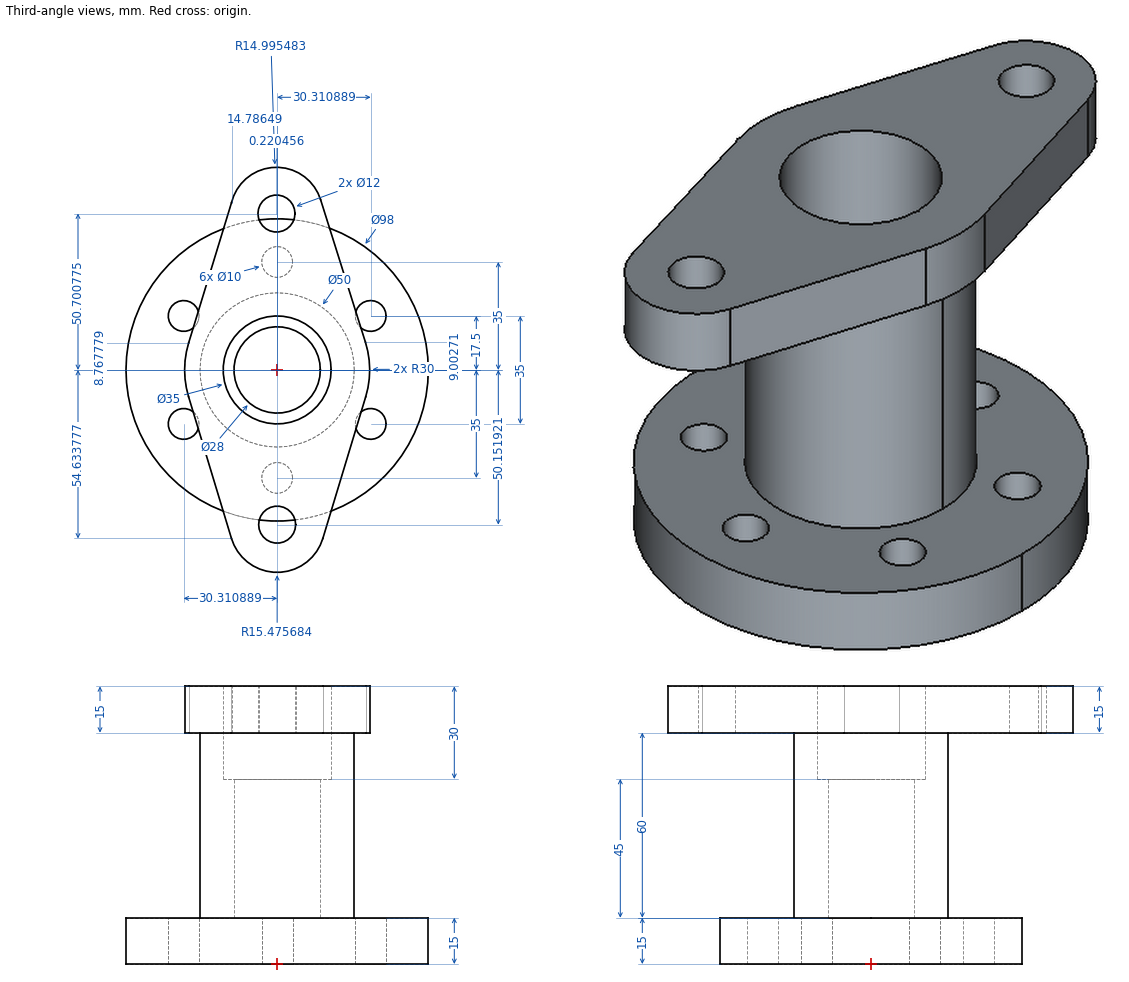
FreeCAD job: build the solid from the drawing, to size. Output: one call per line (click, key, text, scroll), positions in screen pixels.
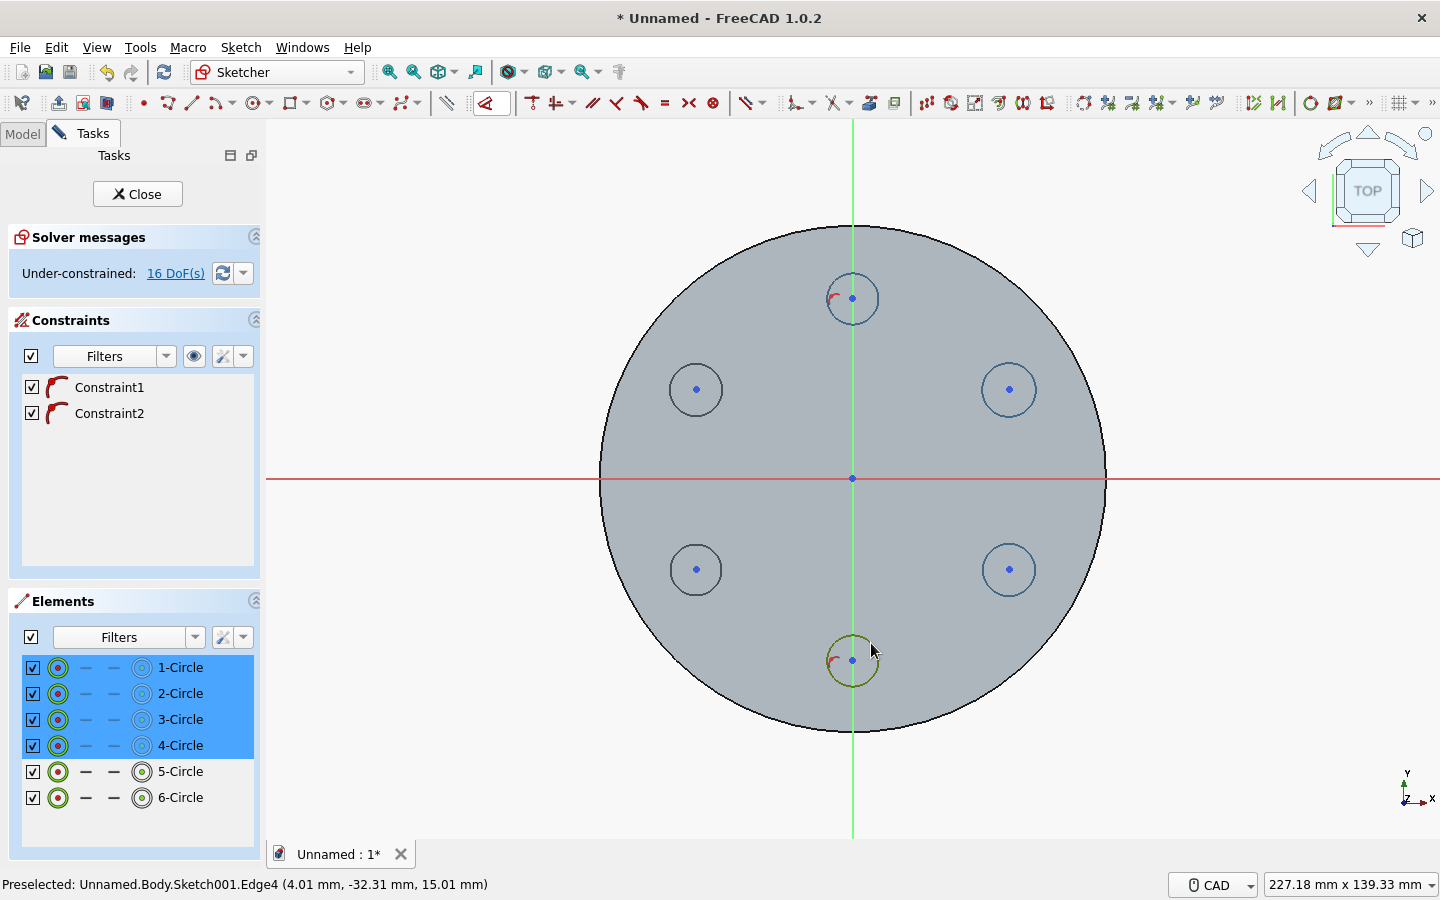
click(714, 552)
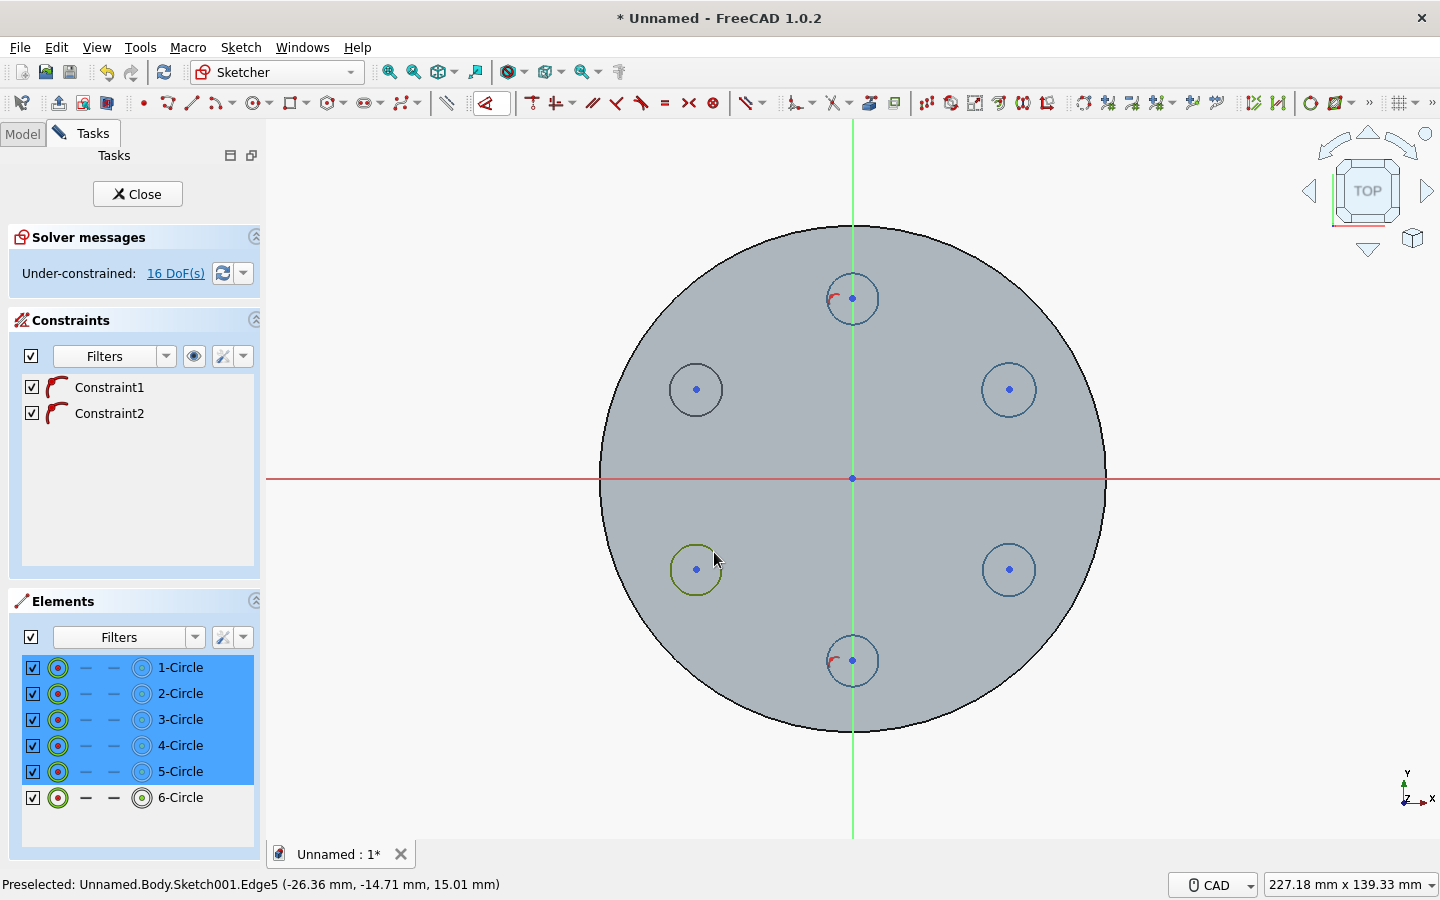
click(714, 371)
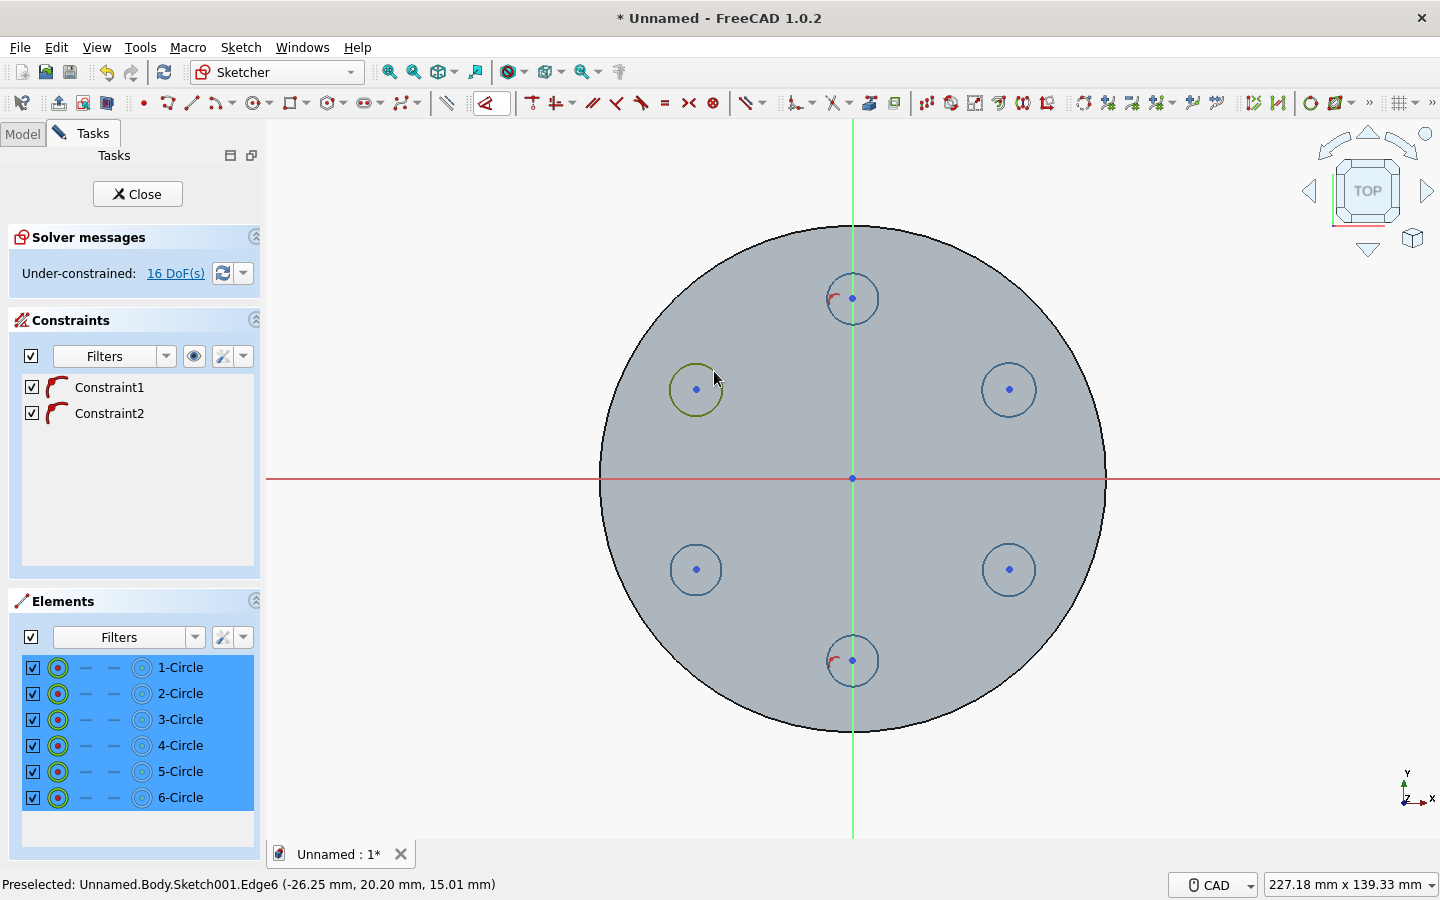
key(e)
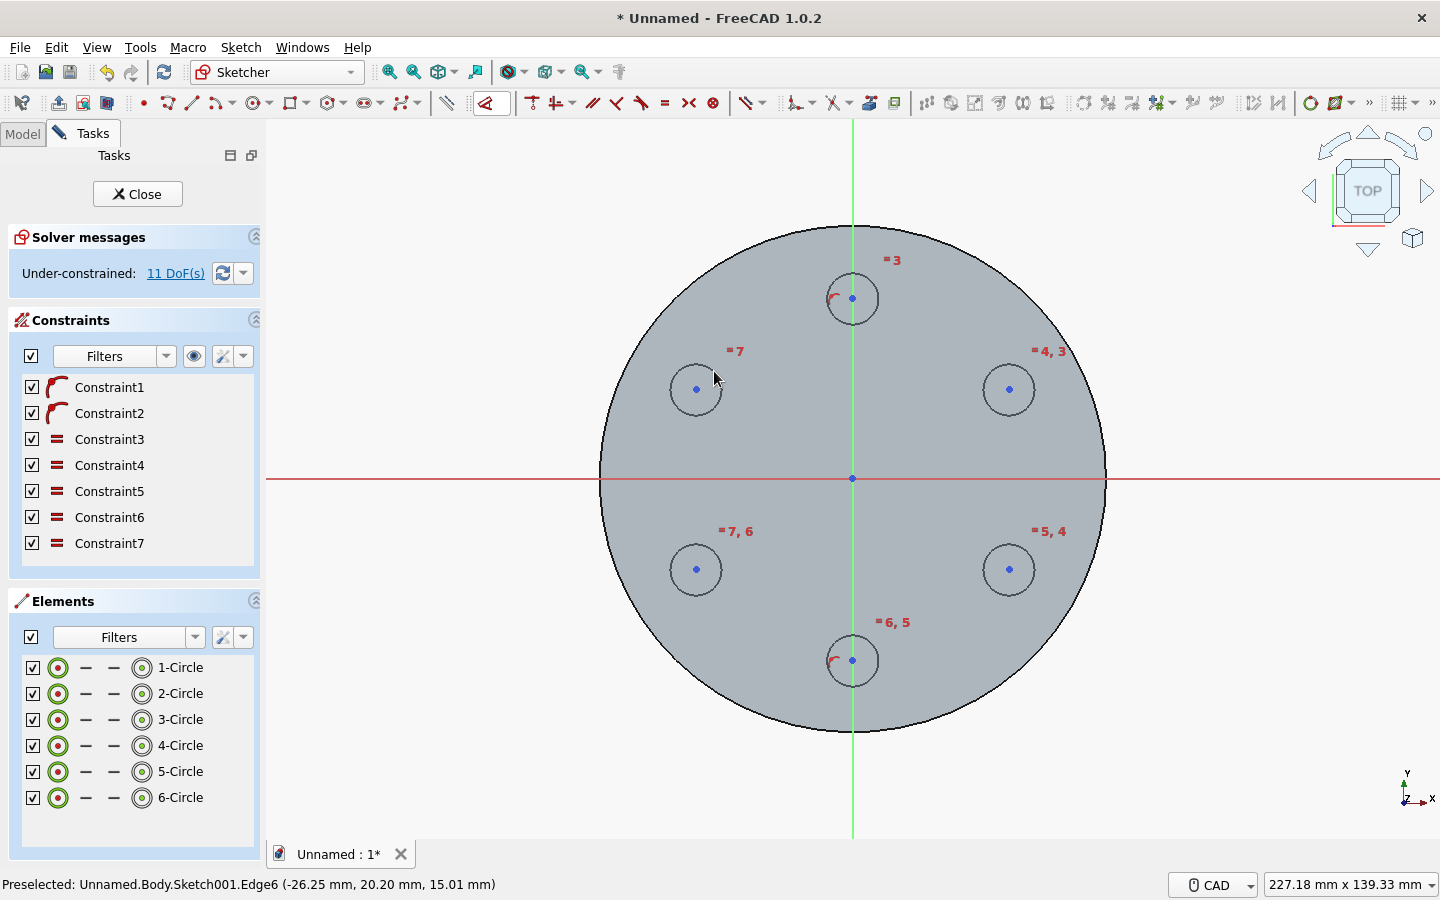
click(1009, 390)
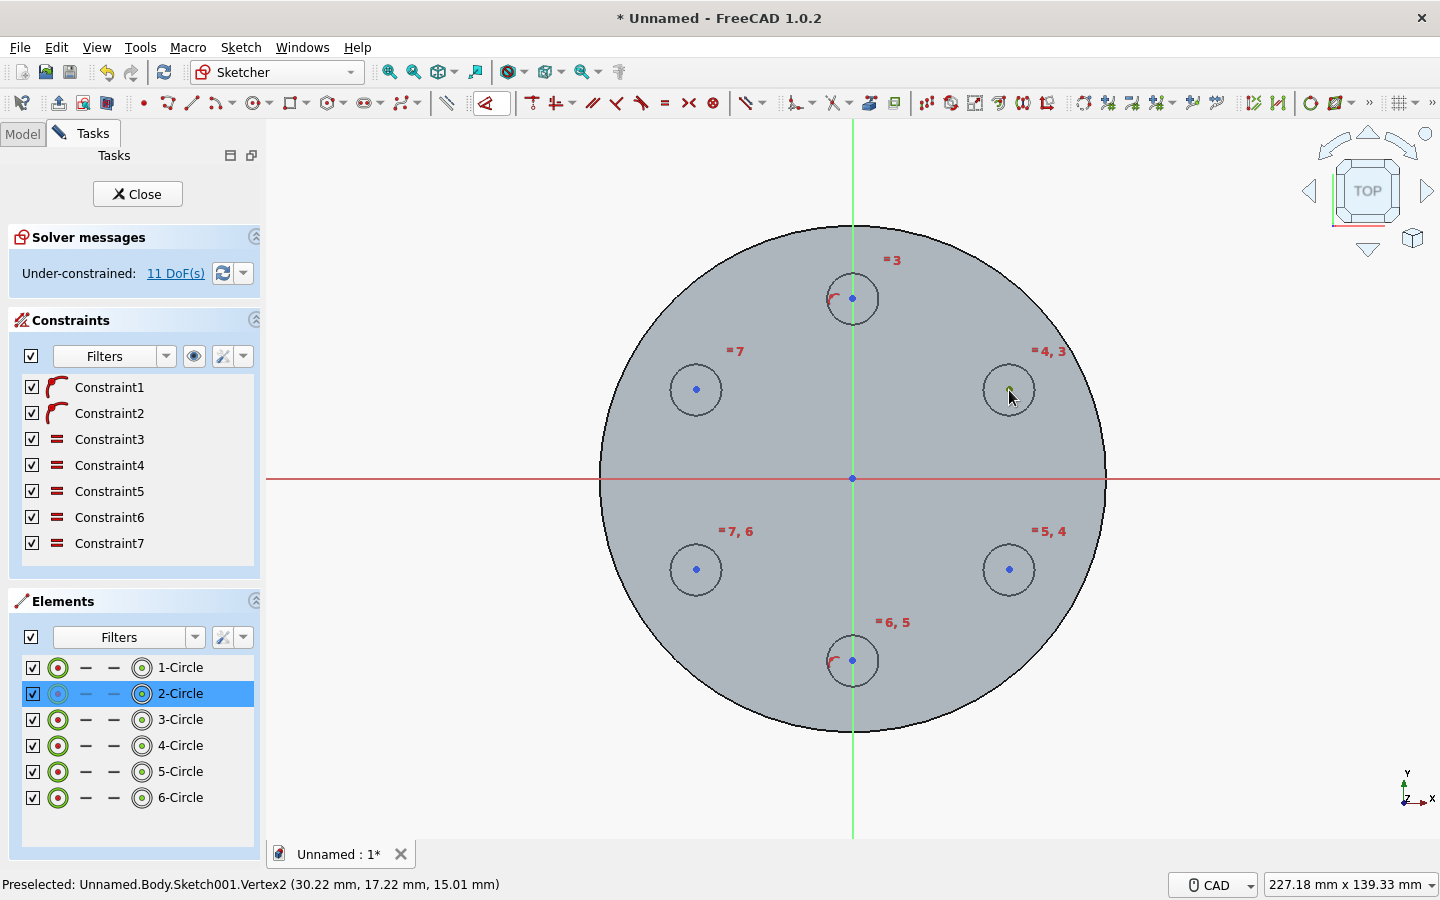
click(1009, 570)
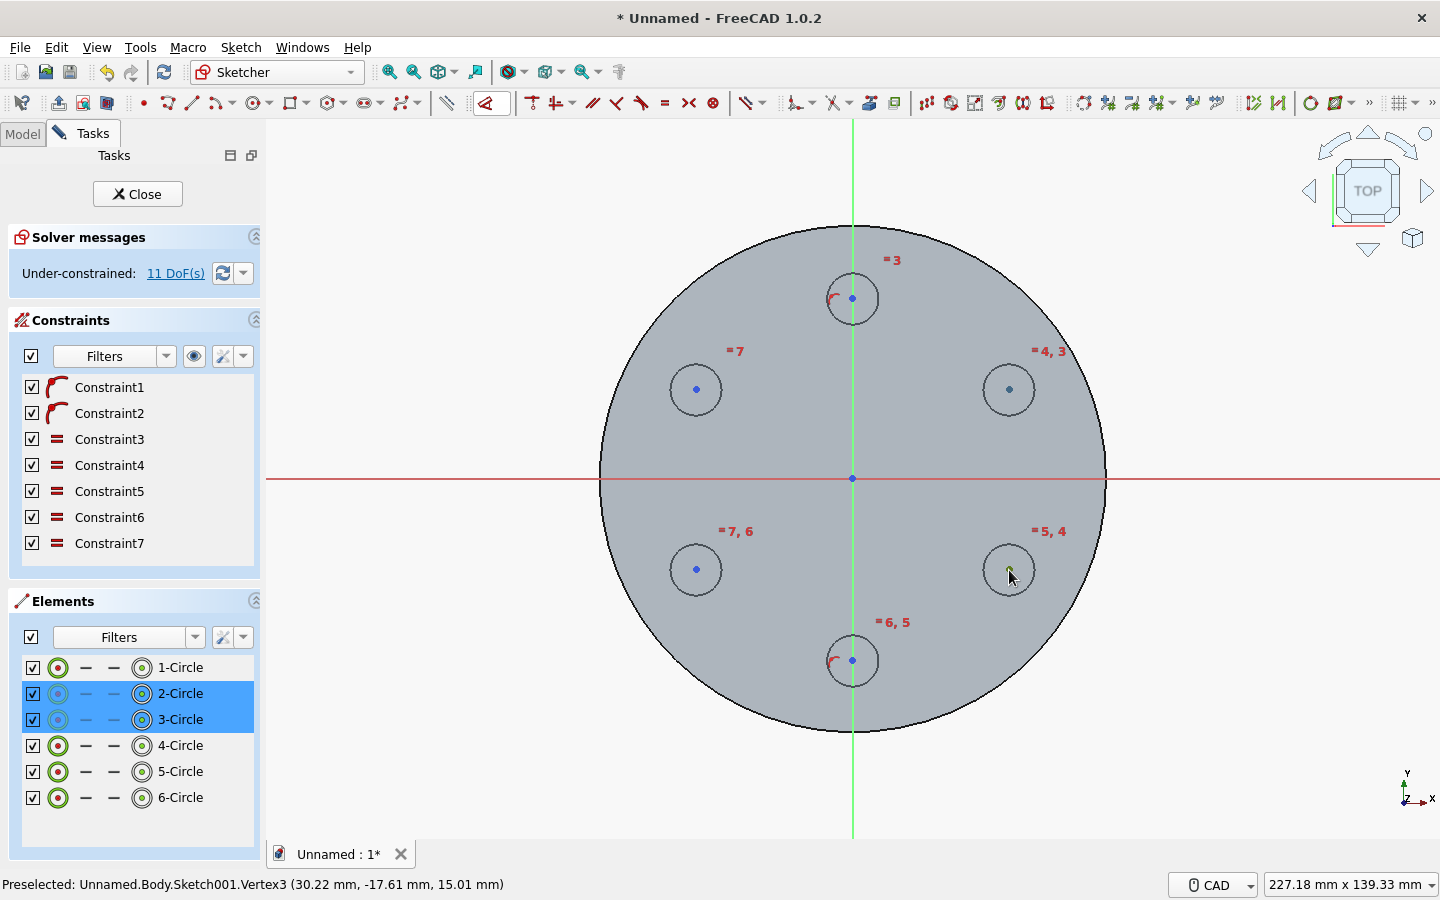
click(574, 104)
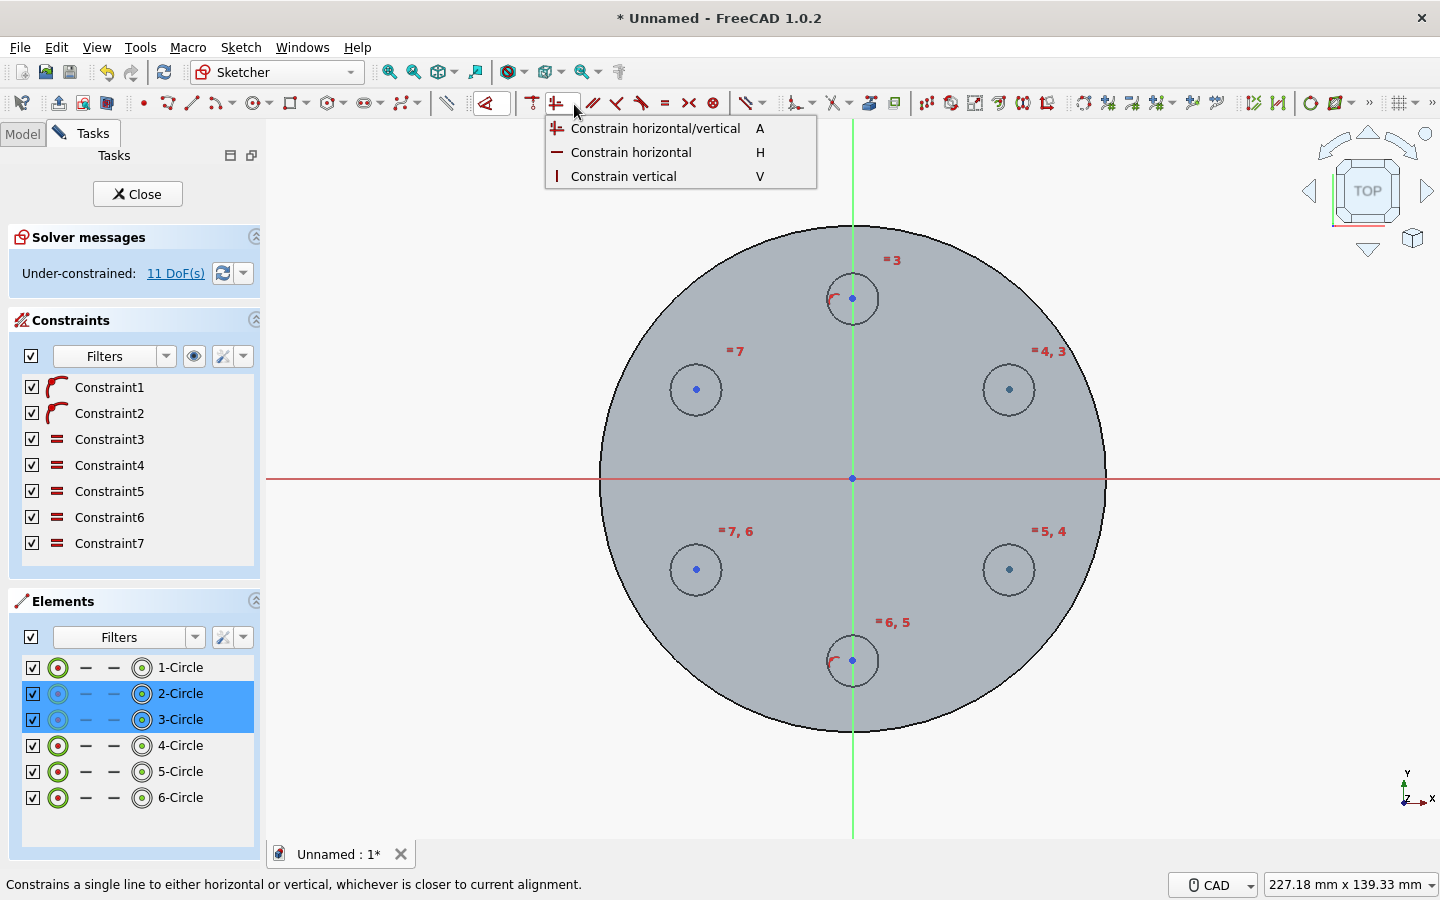
click(681, 176)